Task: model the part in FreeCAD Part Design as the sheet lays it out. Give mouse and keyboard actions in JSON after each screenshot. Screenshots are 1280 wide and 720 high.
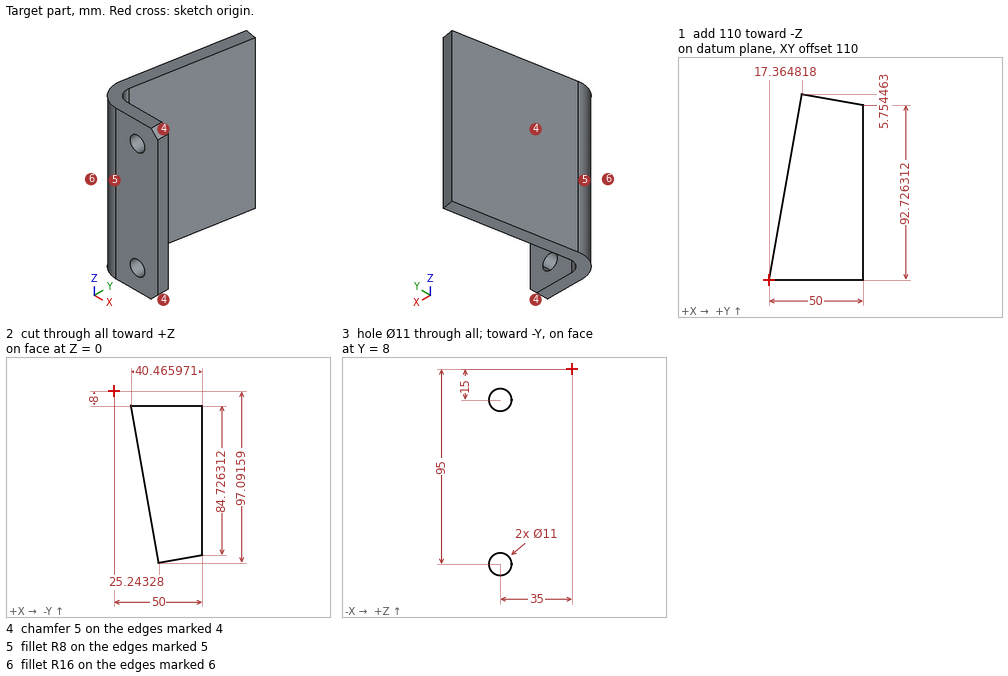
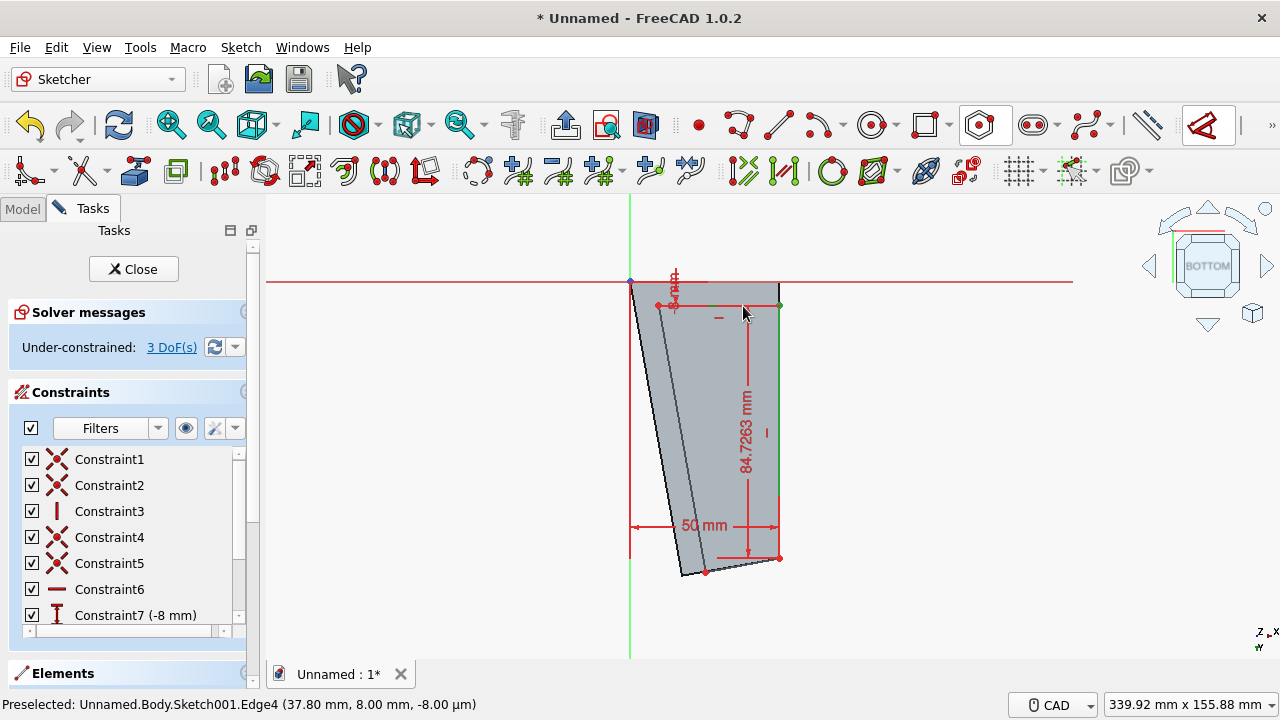
{"action": "left_click", "coordinate": [1230, 126]}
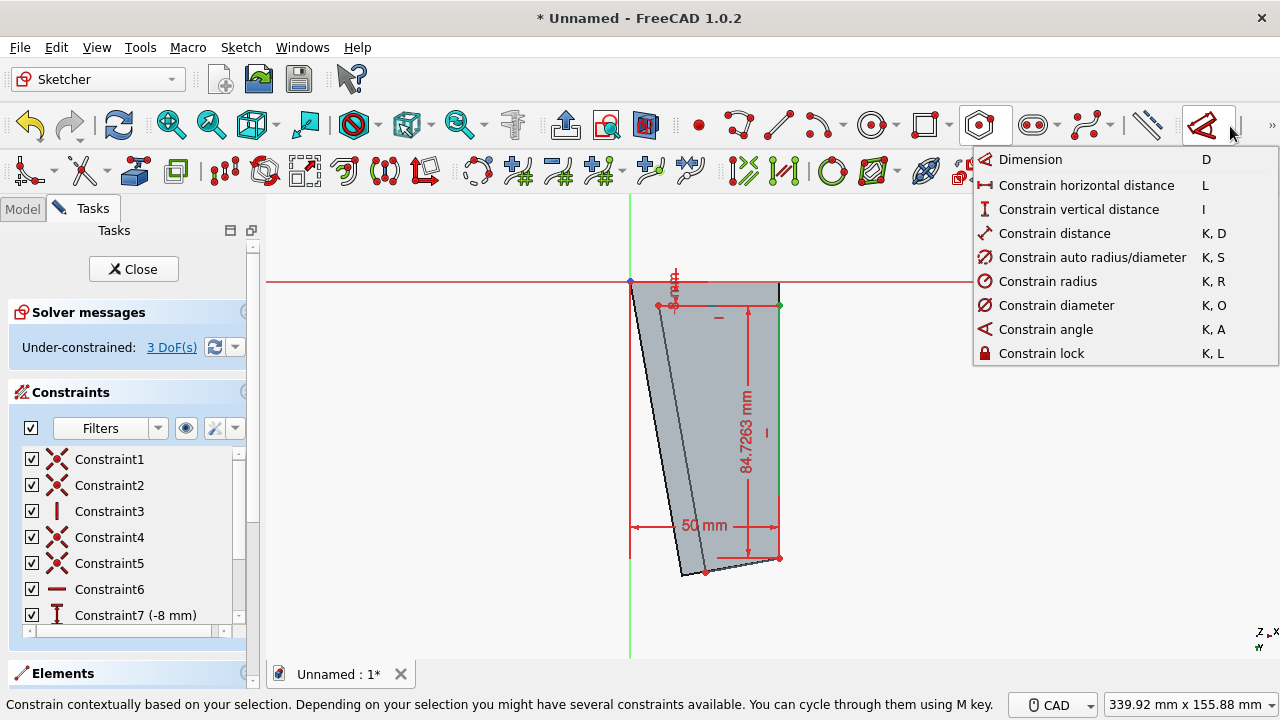
{"action": "left_click", "coordinate": [1126, 185]}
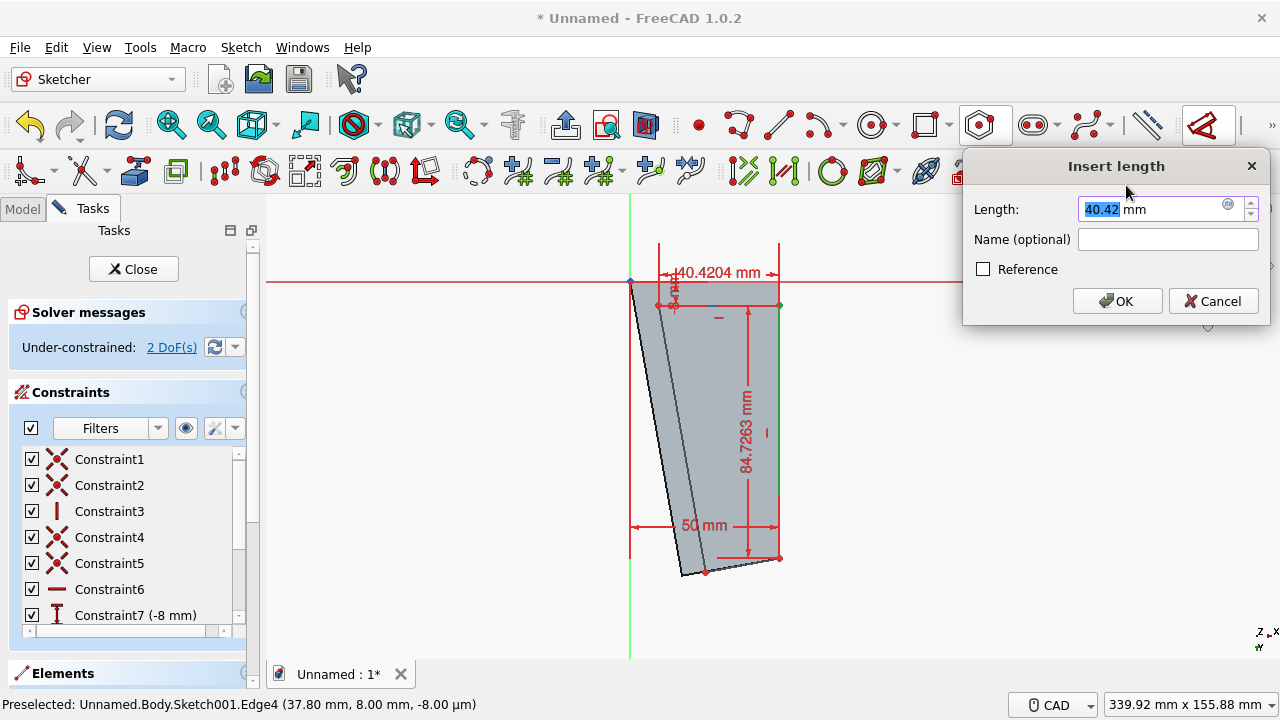
{"action": "type", "text": "40.465971"}
{"action": "key", "text": "Return"}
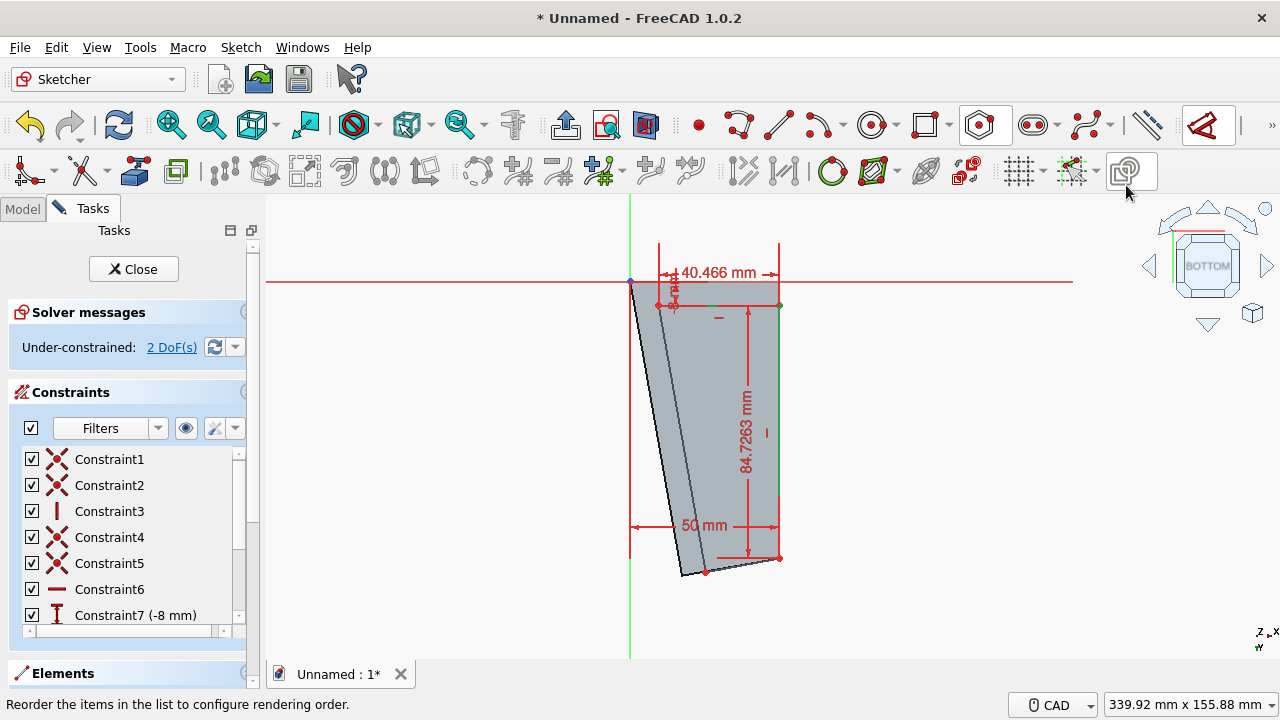
{"action": "left_click", "coordinate": [706, 572]}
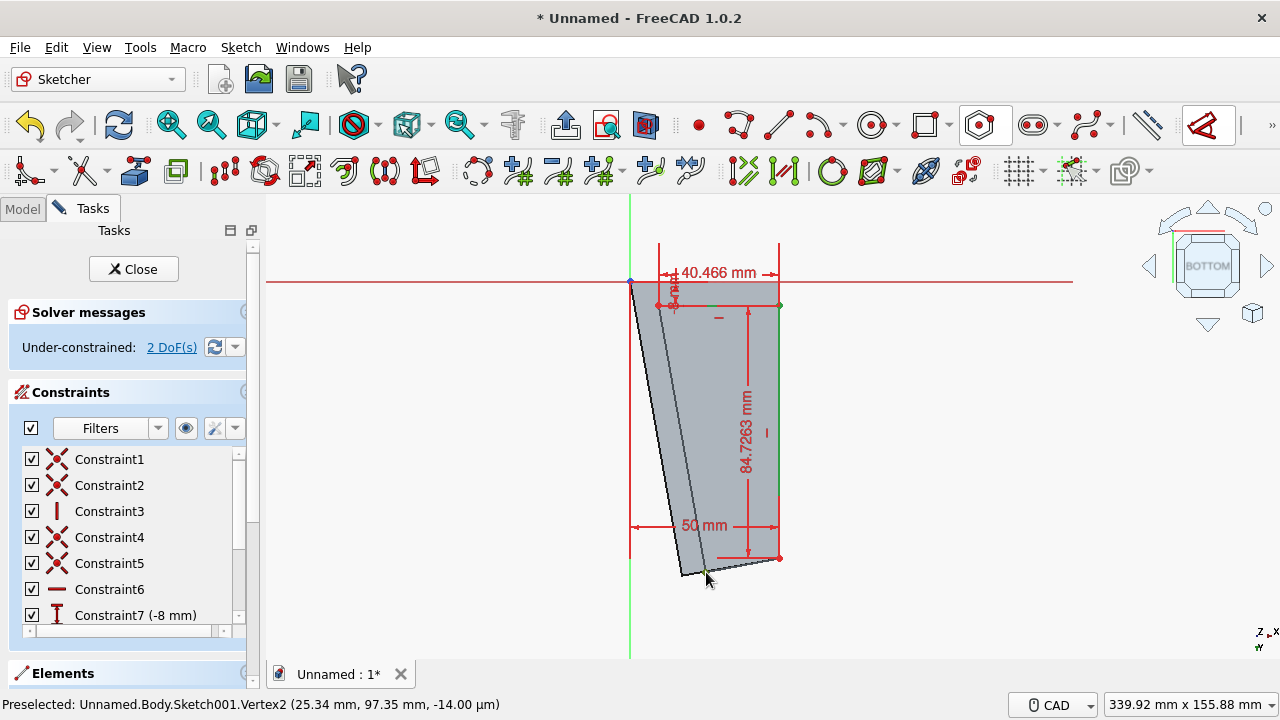
{"action": "key", "text": "l"}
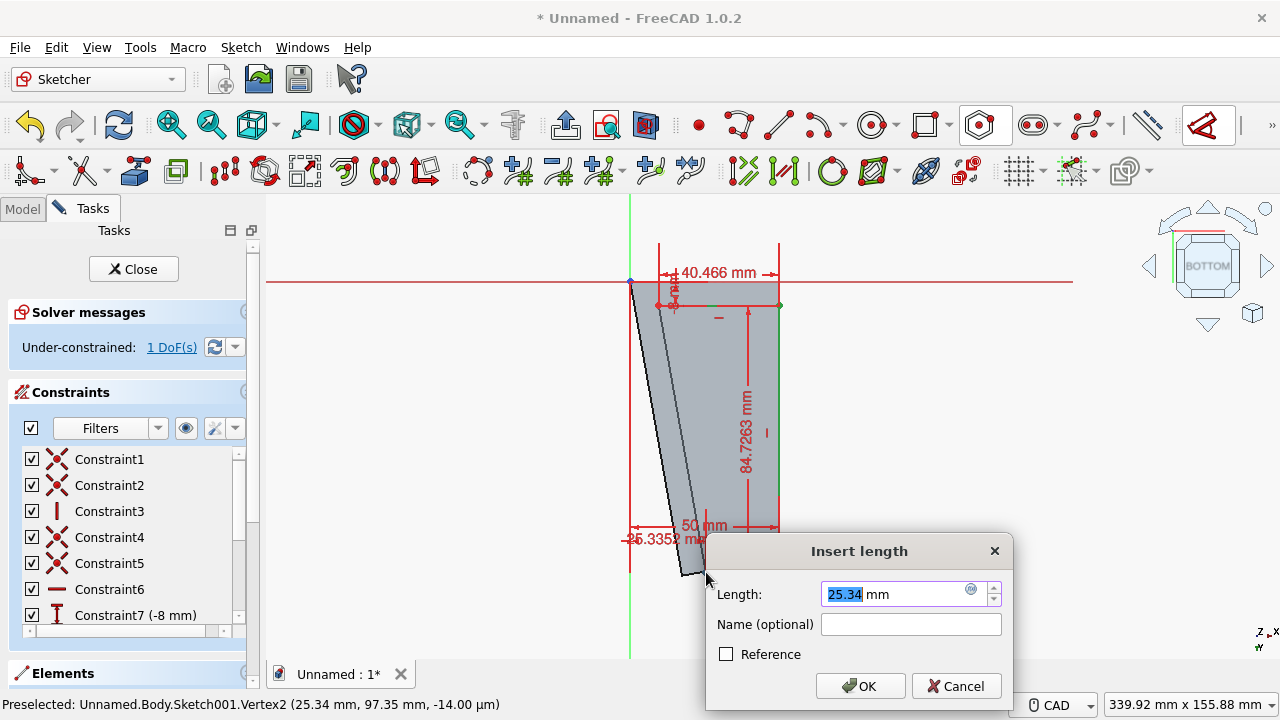
{"action": "type", "text": "25.24328"}
{"action": "key", "text": "Return"}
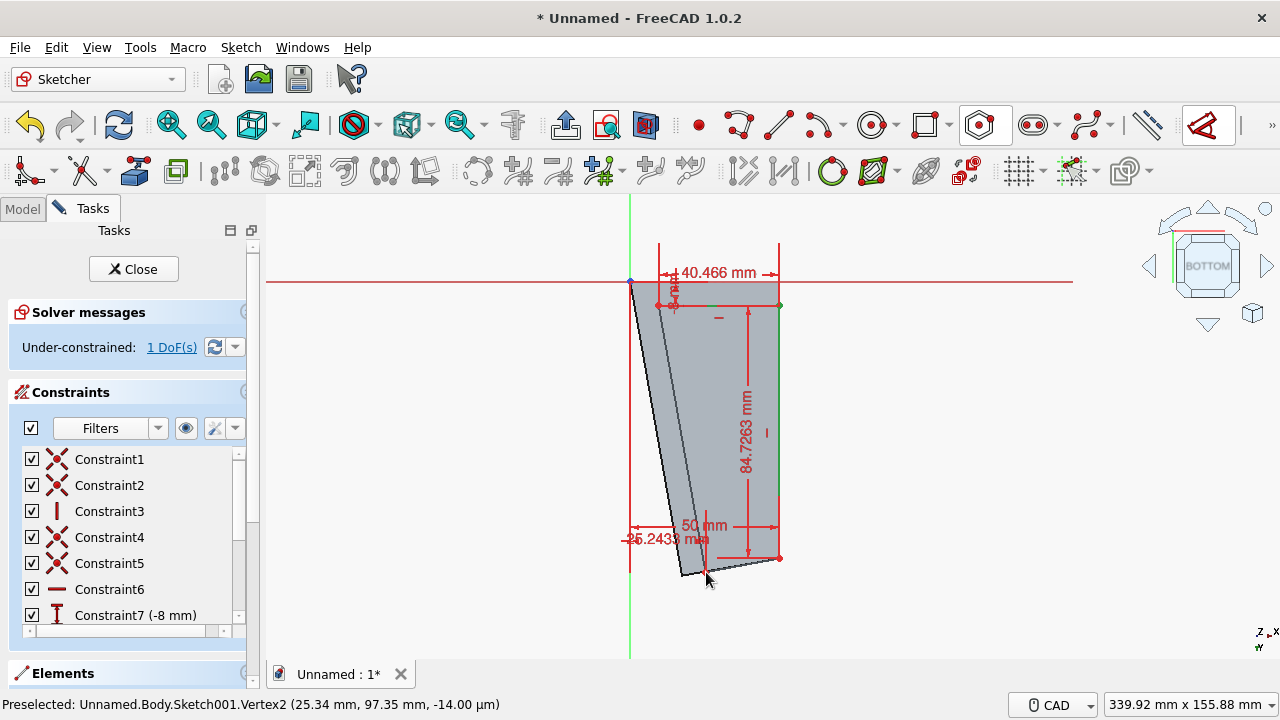
{"action": "left_click", "coordinate": [706, 572]}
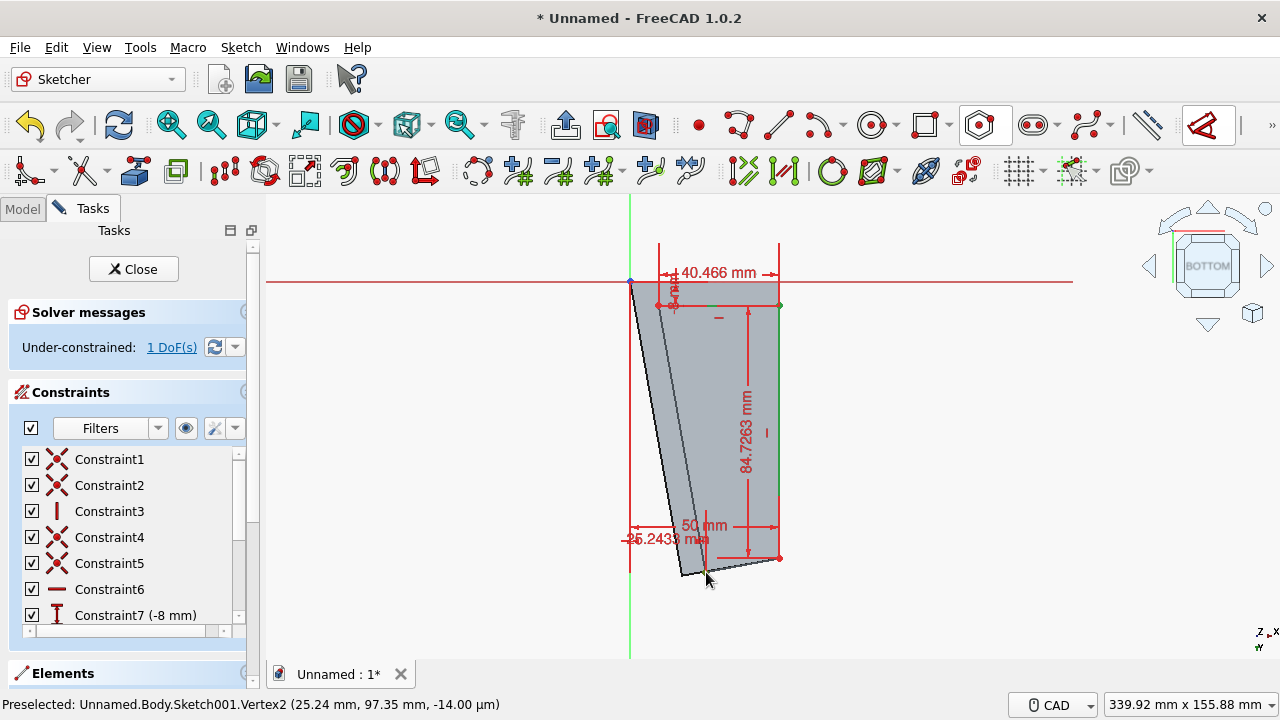
{"action": "left_click", "coordinate": [1230, 126]}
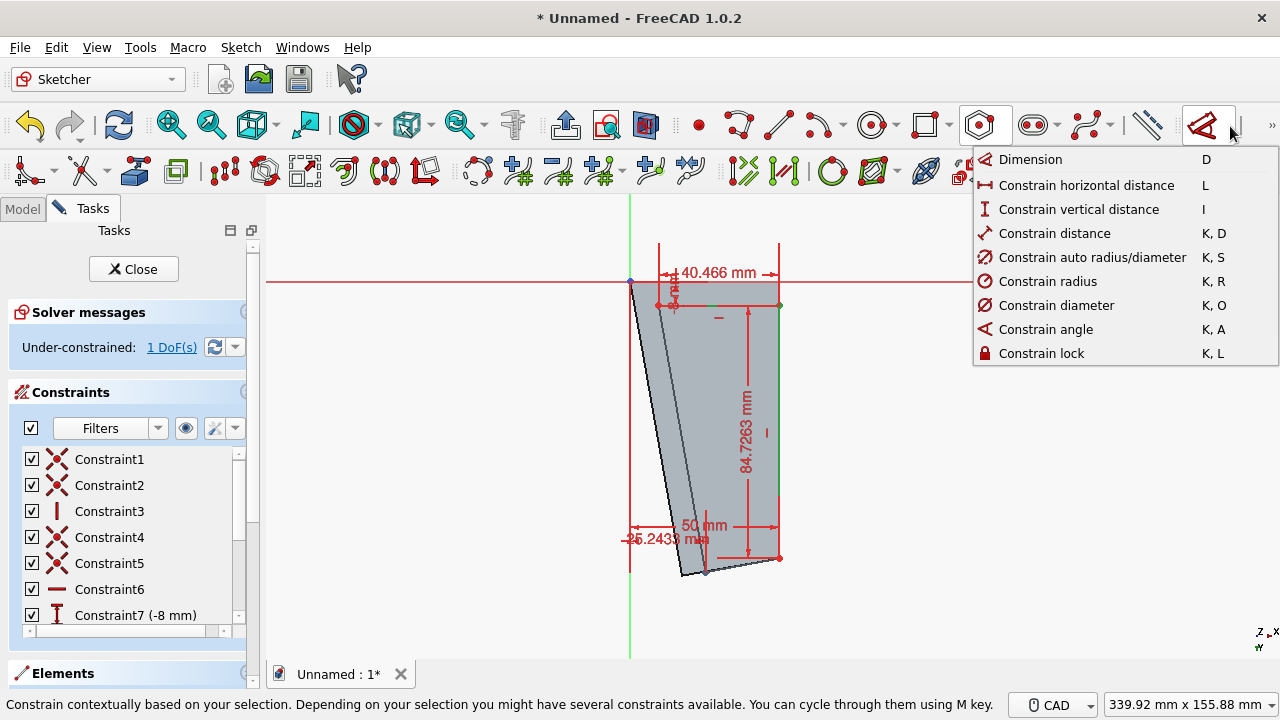
{"action": "left_click", "coordinate": [1126, 209]}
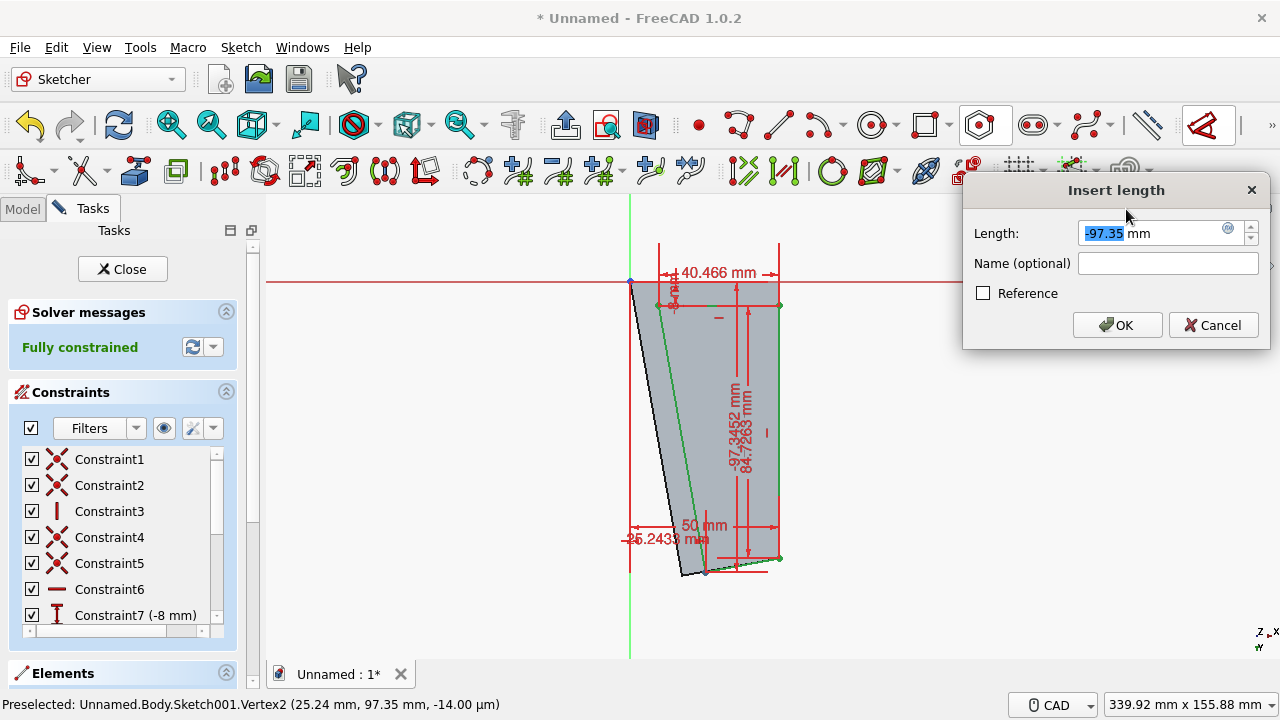
{"action": "type", "text": "-97.09159"}
{"action": "key", "text": "Return"}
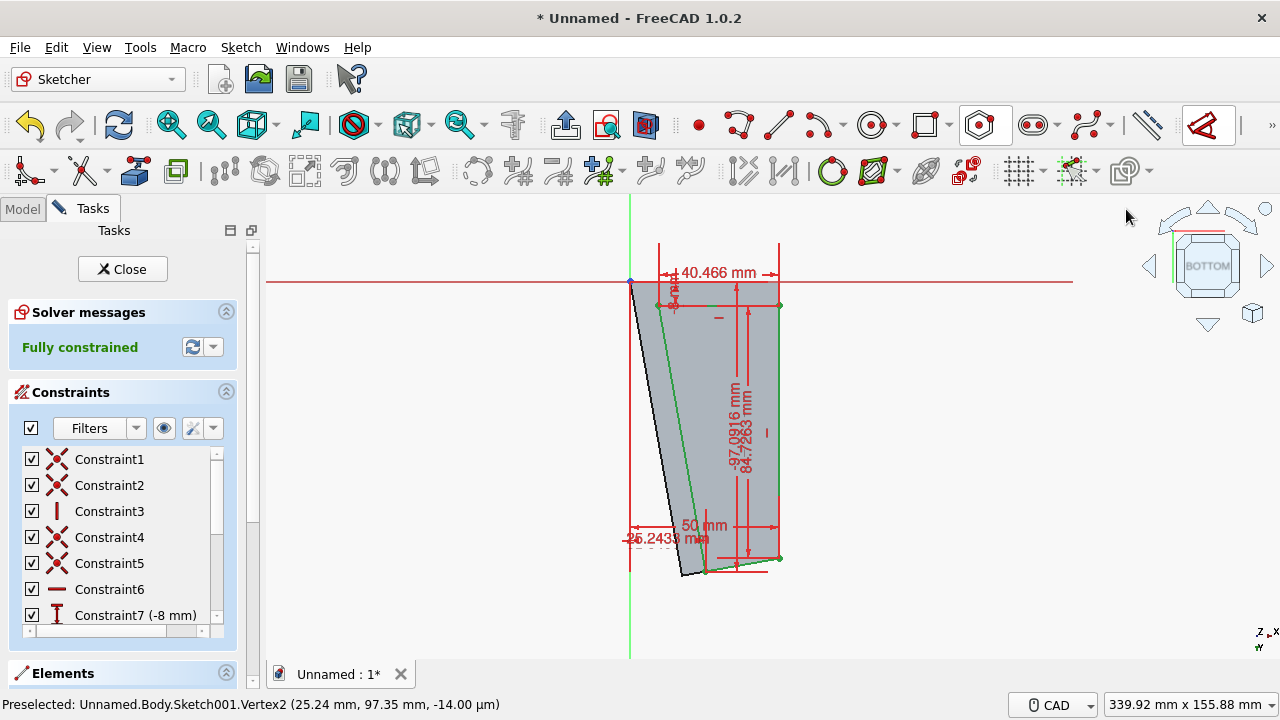
{"action": "left_click", "coordinate": [123, 269]}